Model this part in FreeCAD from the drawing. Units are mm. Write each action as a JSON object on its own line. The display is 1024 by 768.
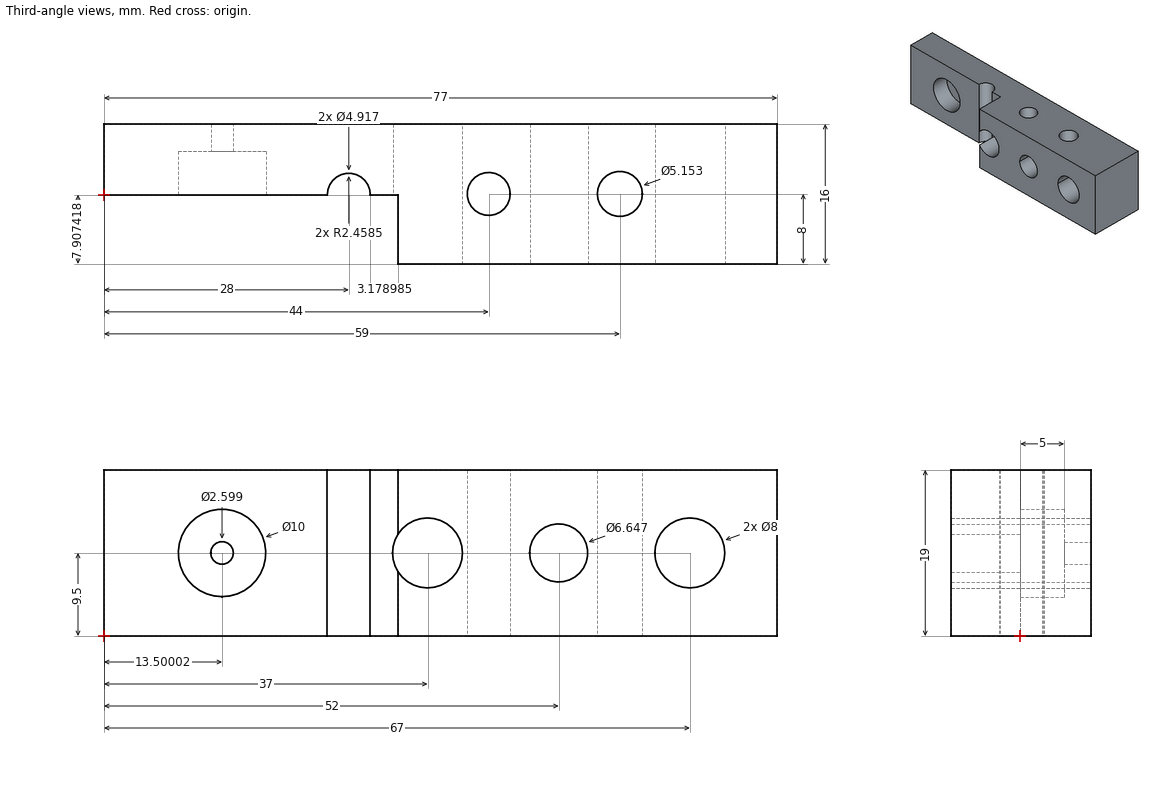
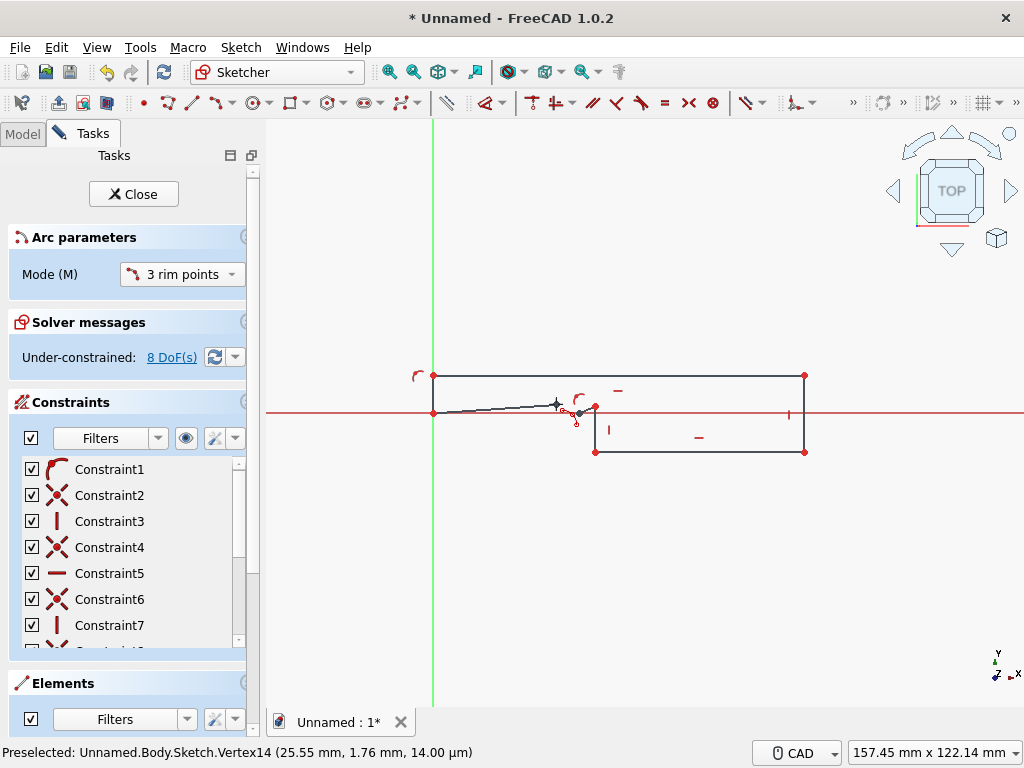
{"action": "left_click", "coordinate": [556, 405]}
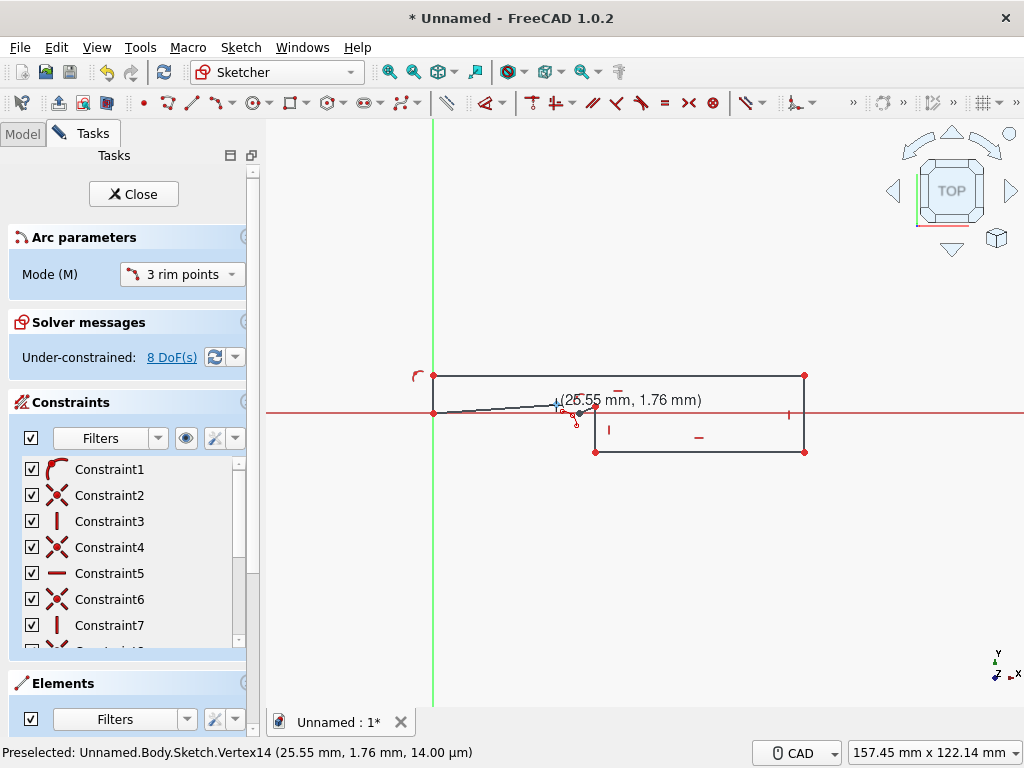
{"action": "scroll", "coordinate": [580, 413], "scroll_direction": "up", "scroll_amount": 4}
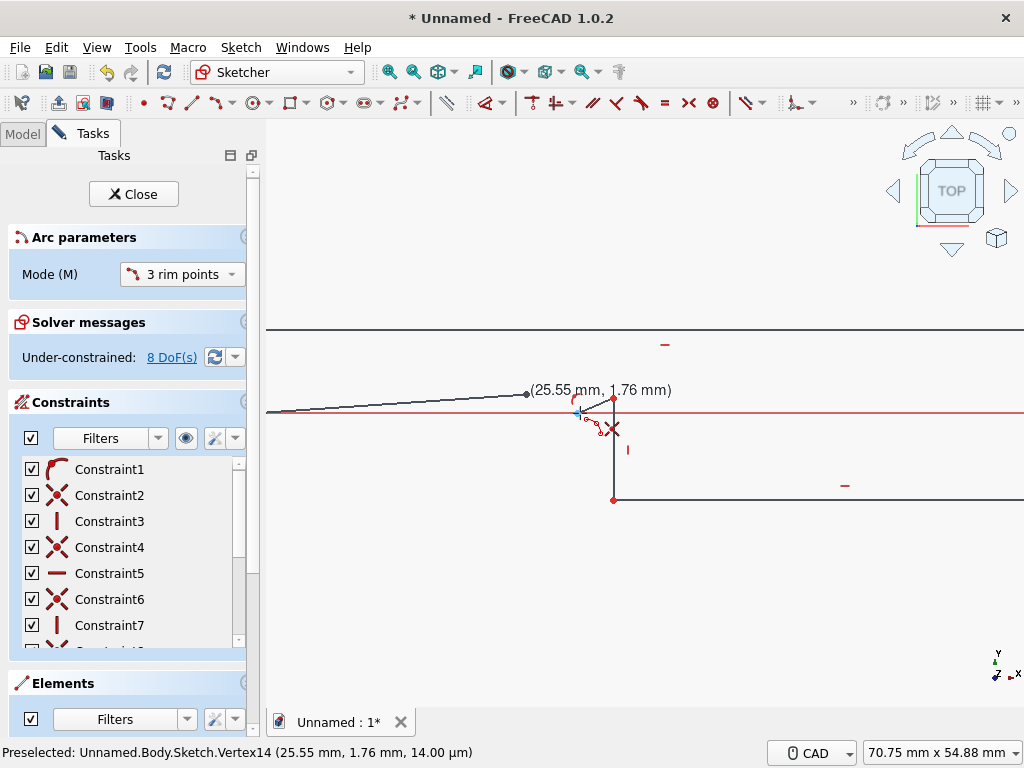
{"action": "left_click", "coordinate": [578, 413]}
{"action": "left_click", "coordinate": [552, 387]}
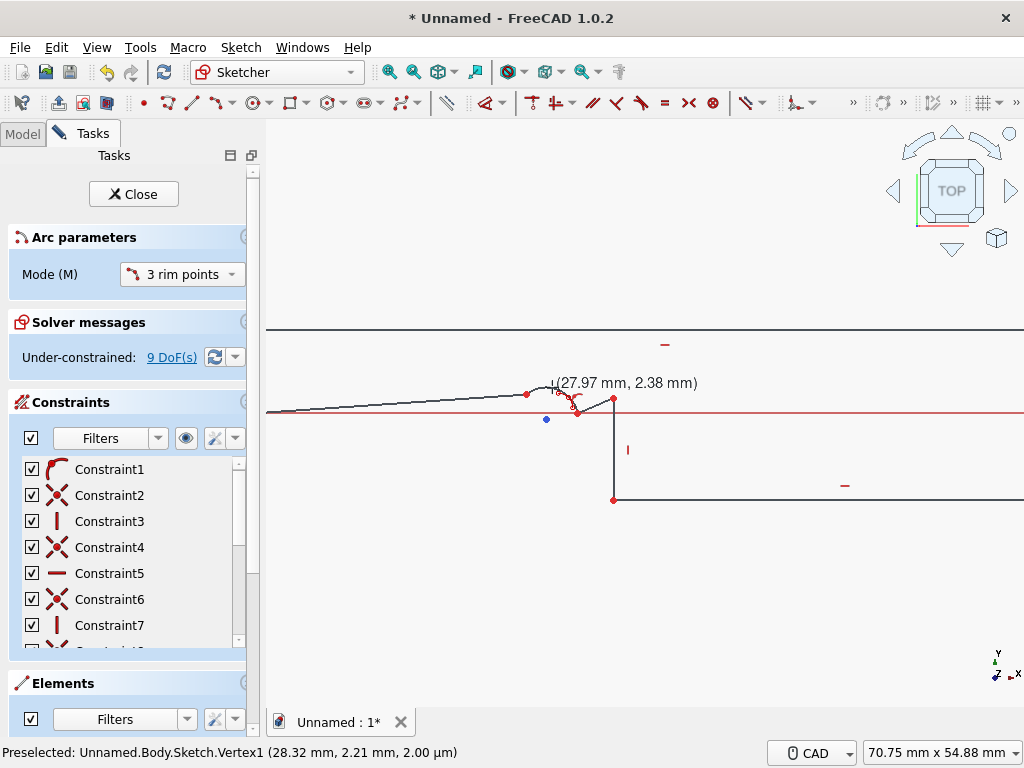
{"action": "left_click", "coordinate": [254, 104]}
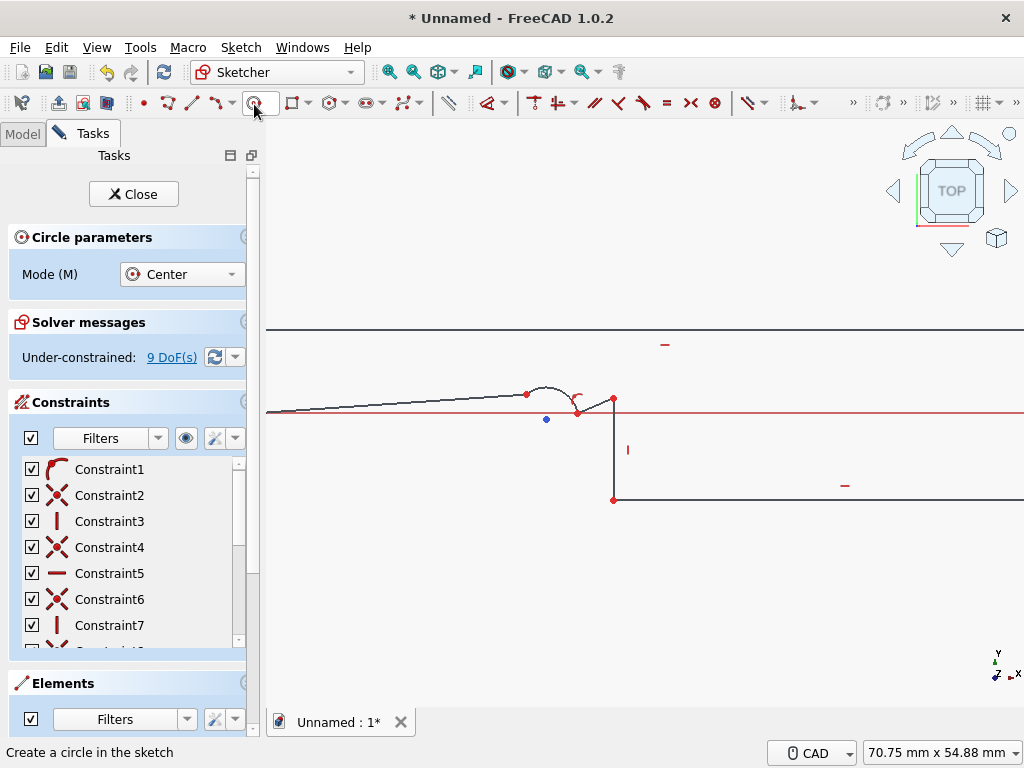
{"action": "scroll", "coordinate": [724, 412], "scroll_direction": "up", "scroll_amount": 14}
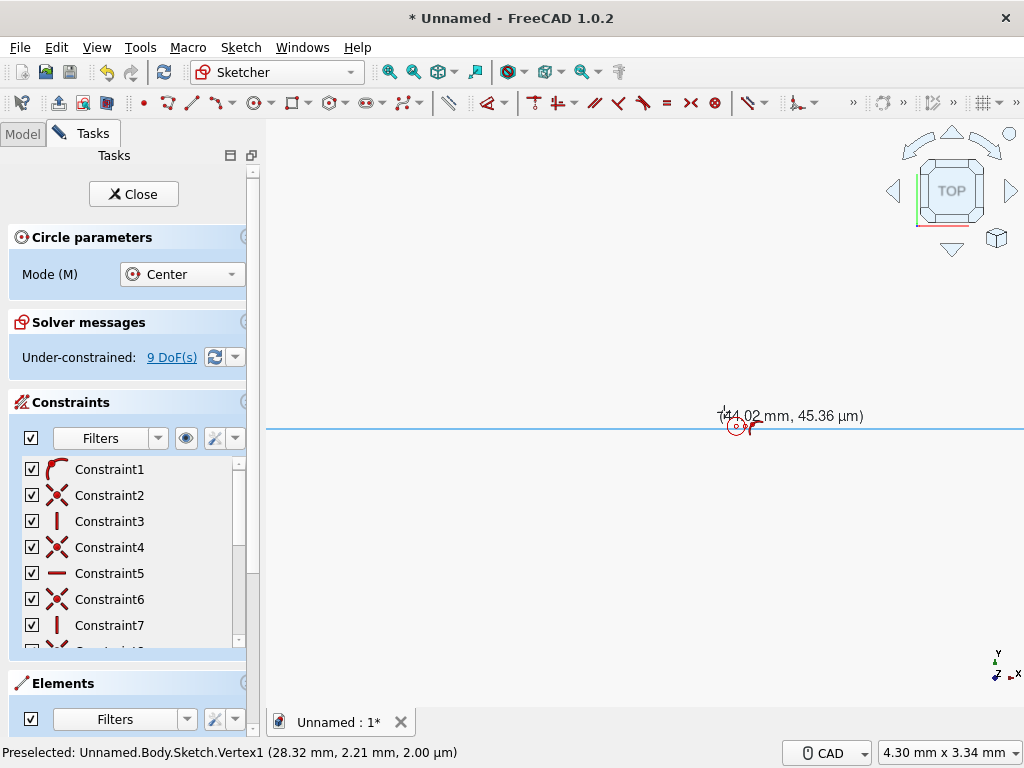
{"action": "left_click", "coordinate": [711, 412]}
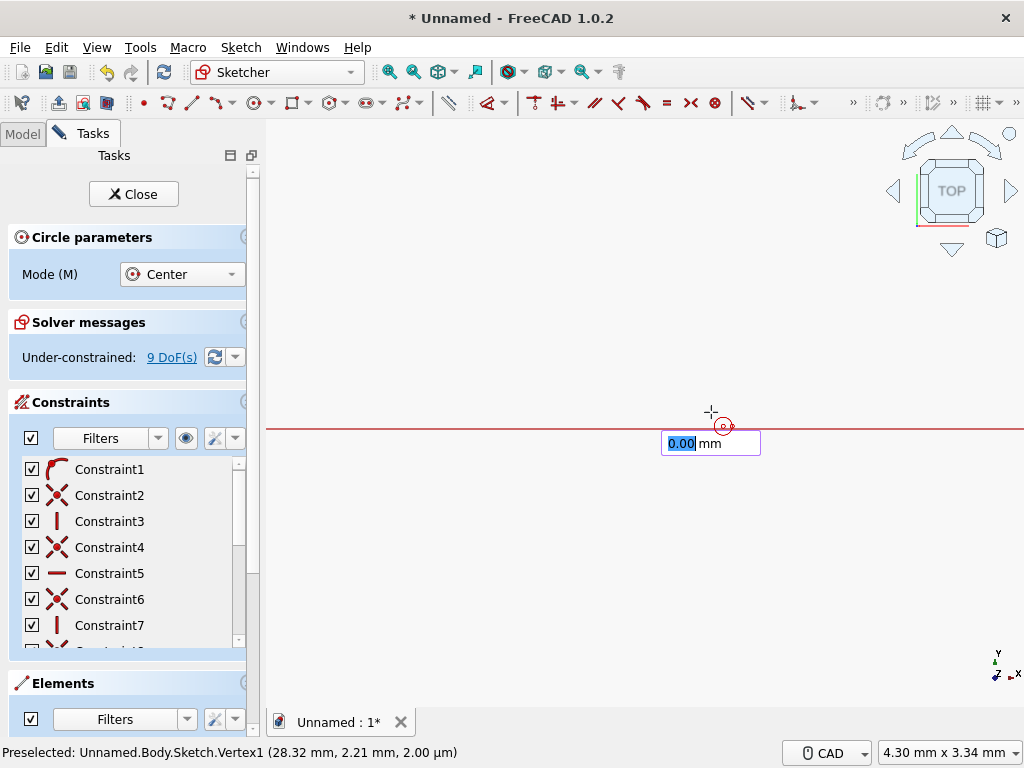
{"action": "scroll", "coordinate": [605, 413], "scroll_direction": "down", "scroll_amount": 17}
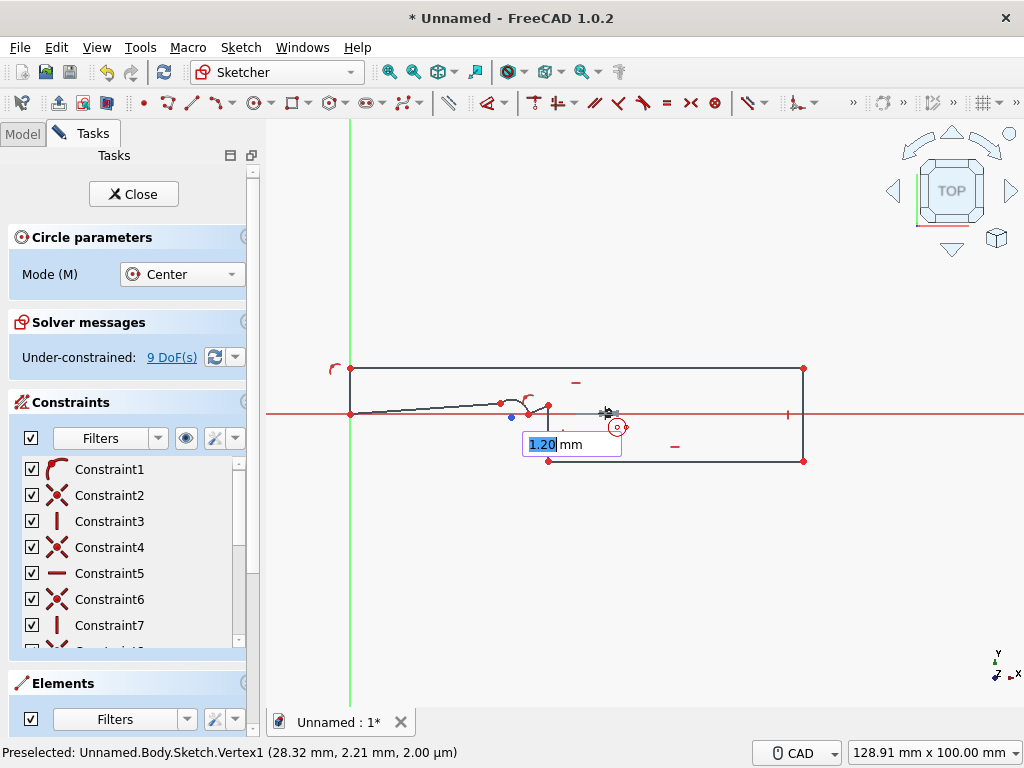
{"action": "scroll", "coordinate": [619, 403], "scroll_direction": "up", "scroll_amount": 2}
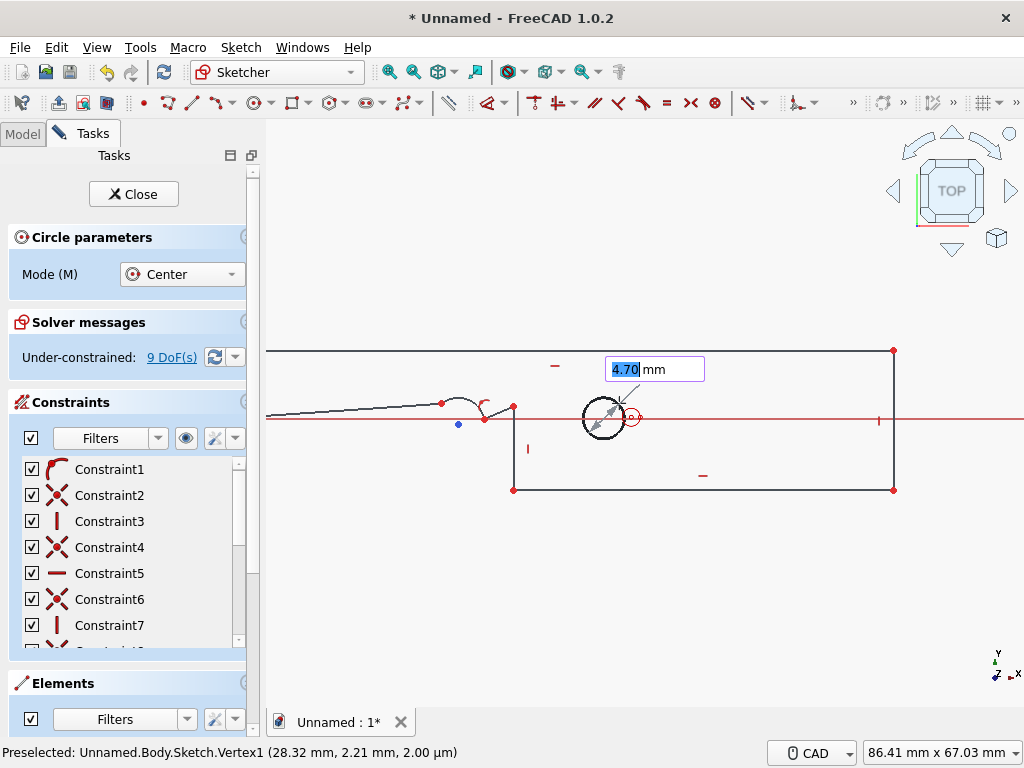
{"action": "left_click", "coordinate": [619, 403]}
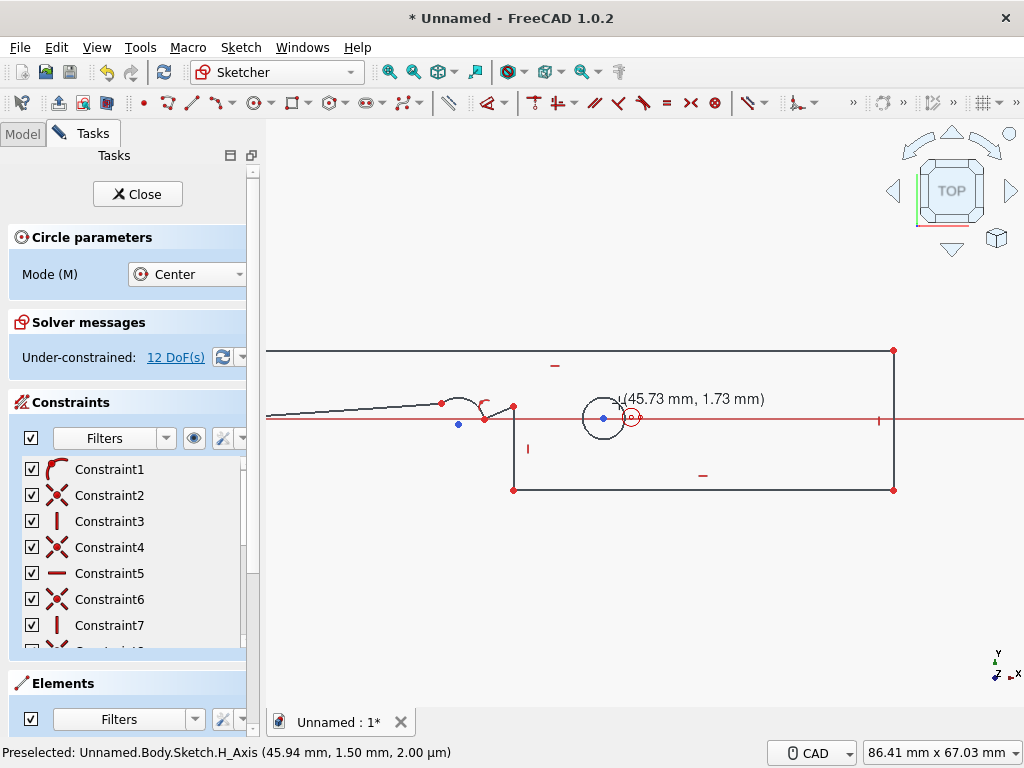
{"action": "scroll", "coordinate": [735, 418], "scroll_direction": "up", "scroll_amount": 15}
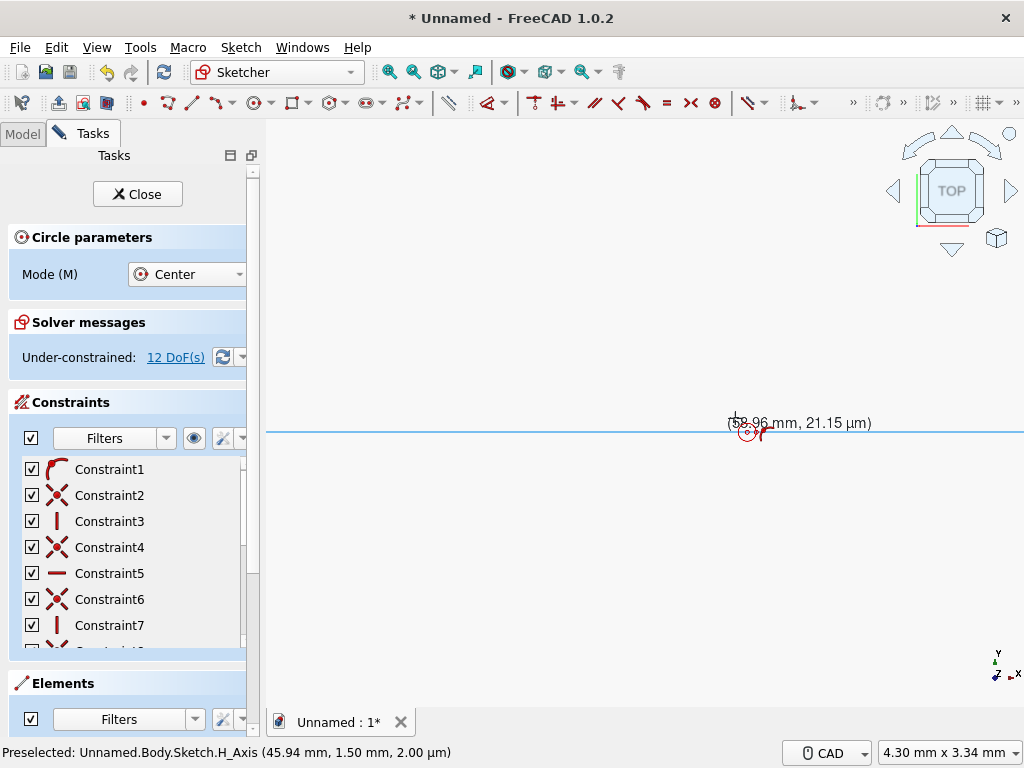
{"action": "left_click", "coordinate": [731, 416]}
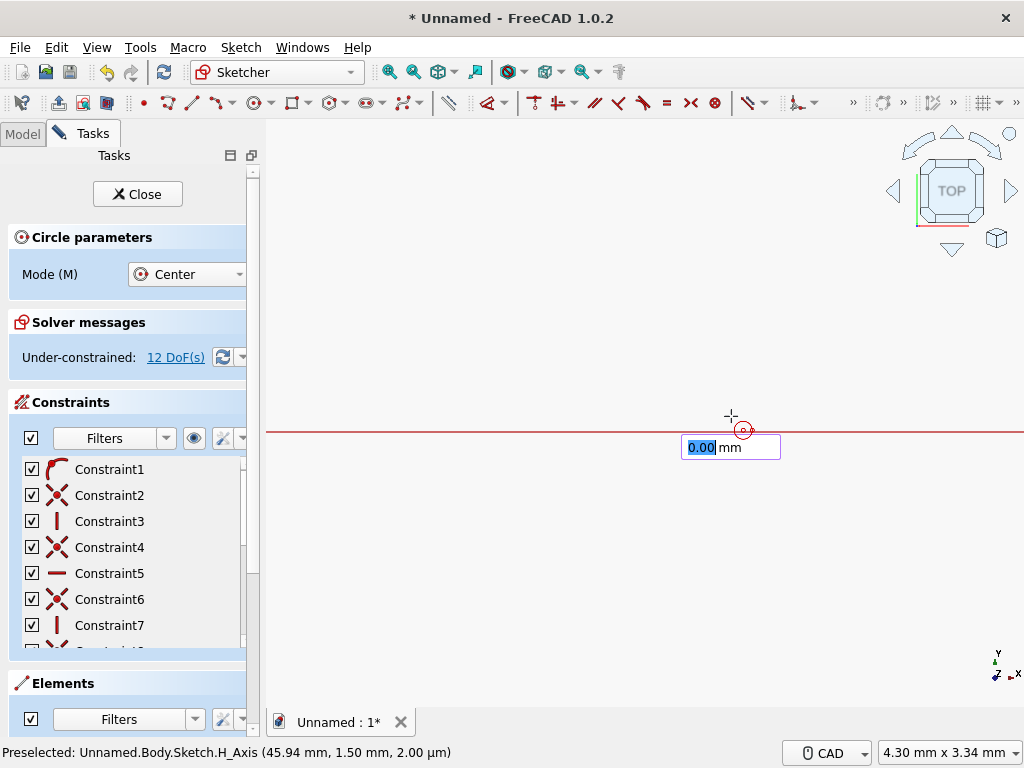
{"action": "scroll", "coordinate": [696, 413], "scroll_direction": "down", "scroll_amount": 17}